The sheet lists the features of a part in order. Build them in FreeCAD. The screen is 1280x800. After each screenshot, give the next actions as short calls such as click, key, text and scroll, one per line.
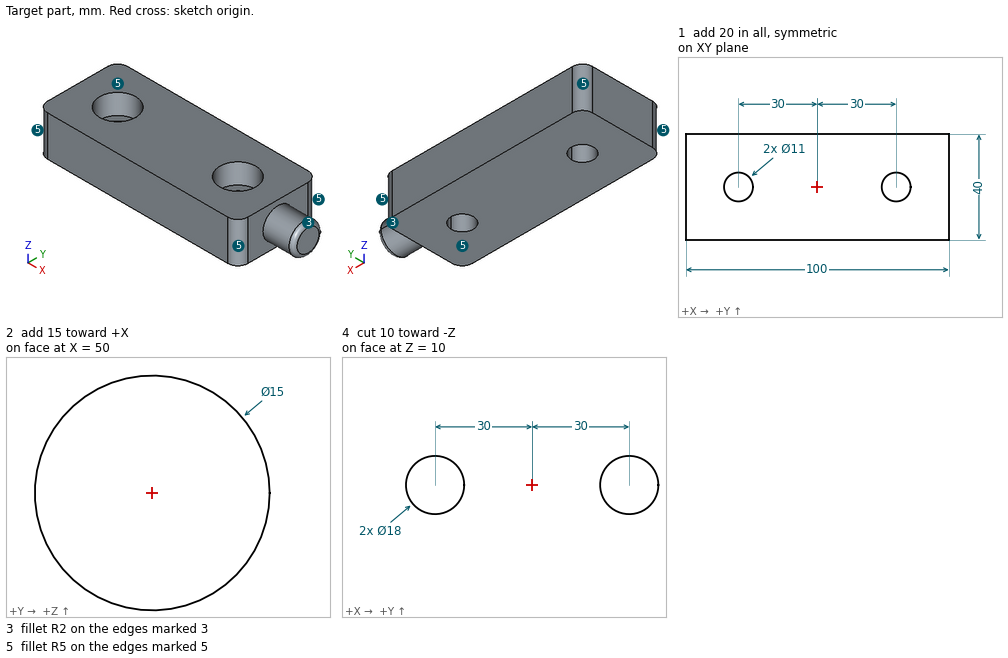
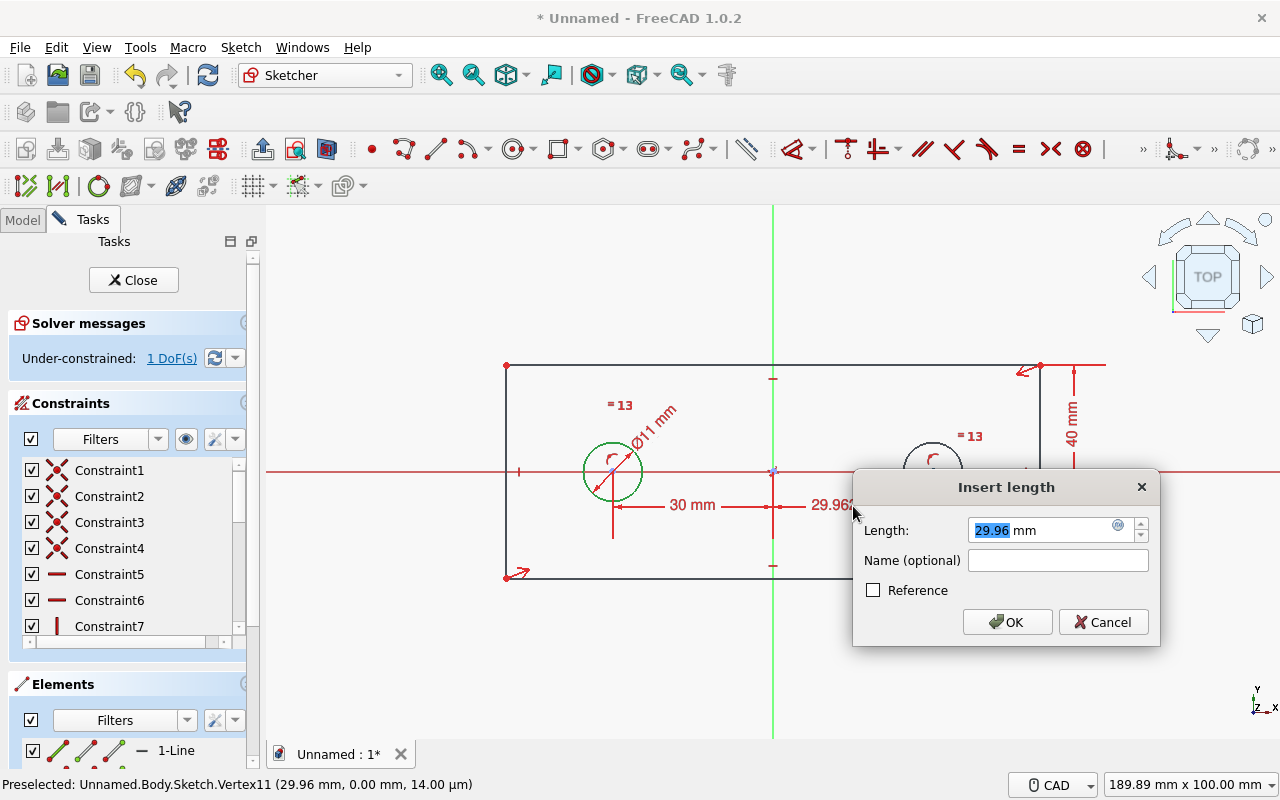
text(30)
key(Return)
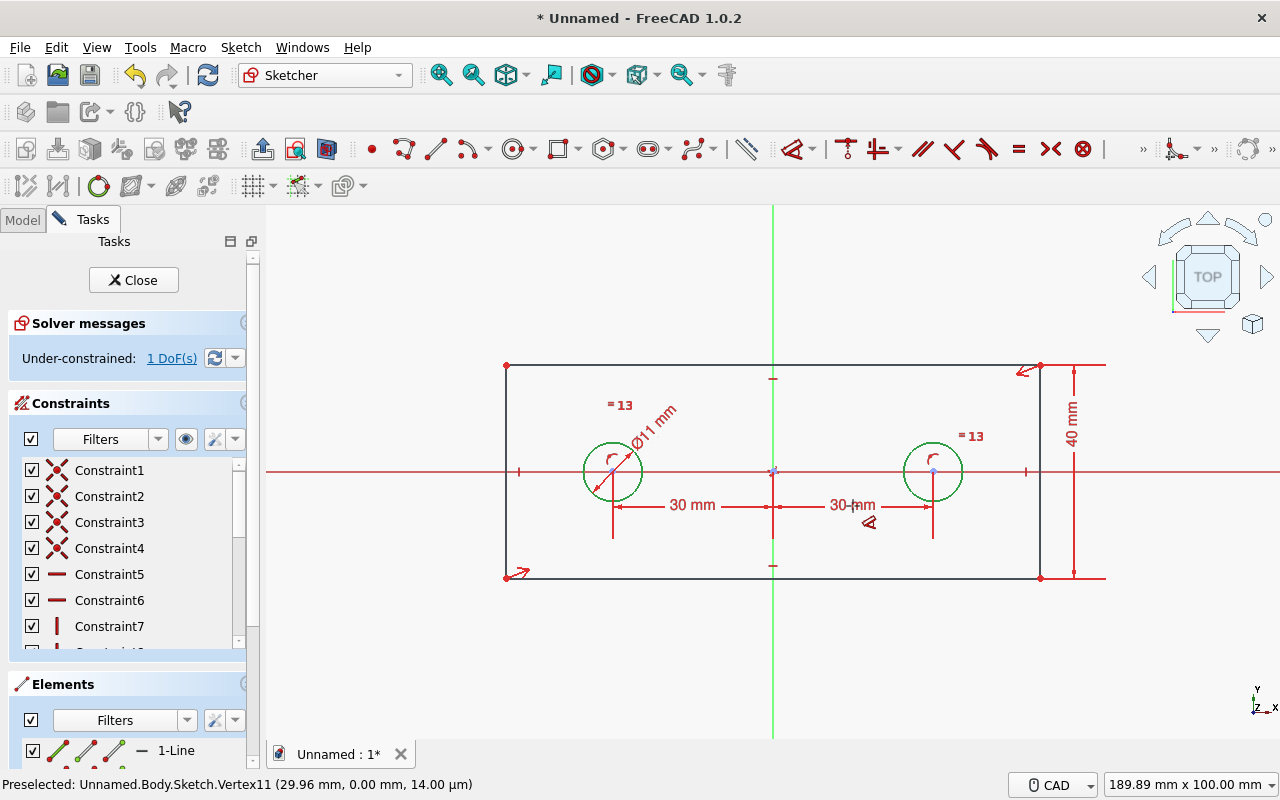
click(666, 579)
click(650, 613)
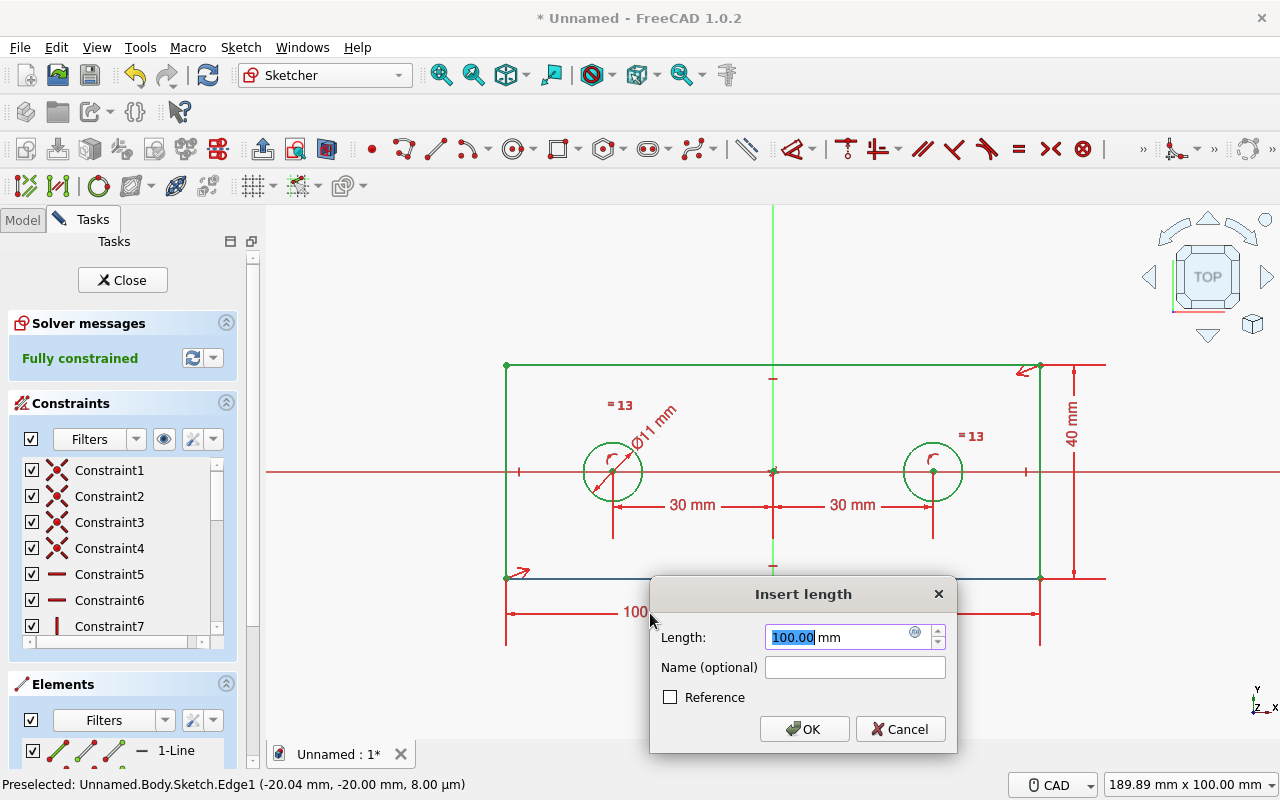
text(100)
key(Return)
key(Escape)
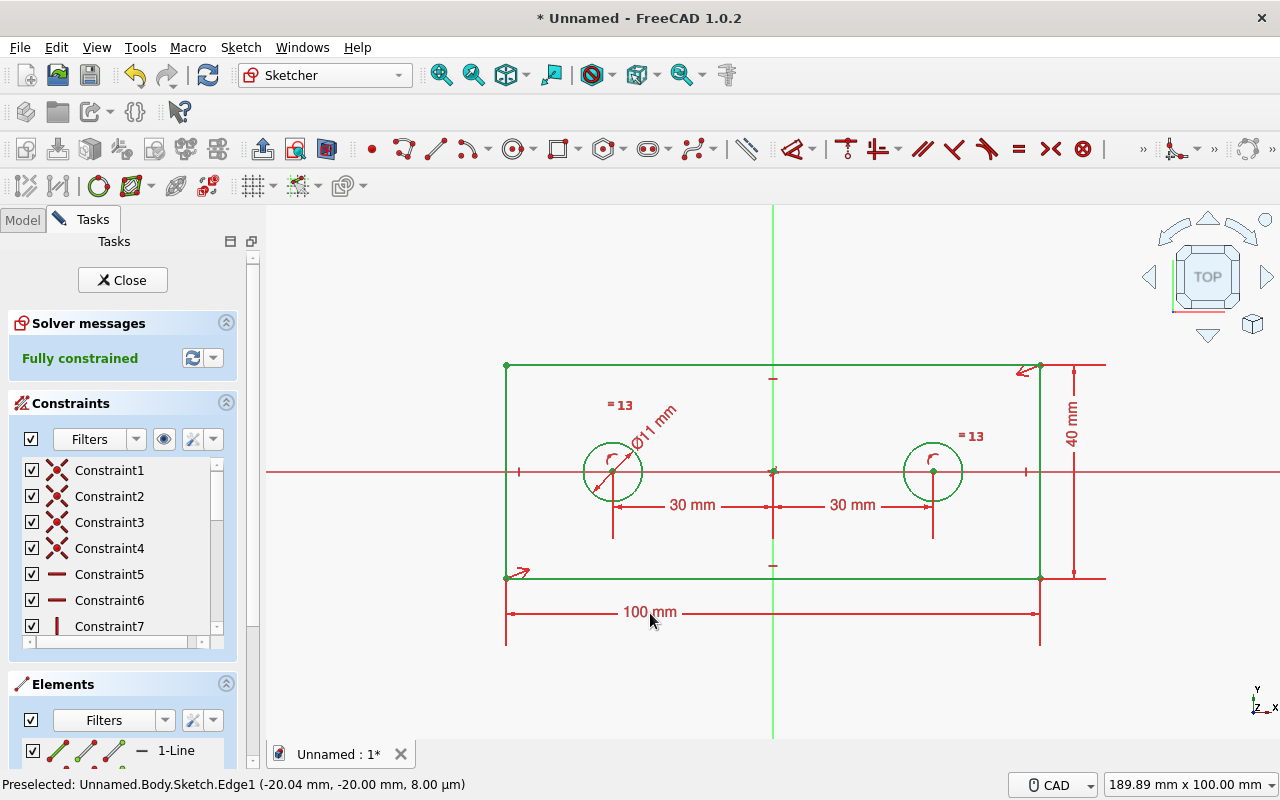
click(123, 280)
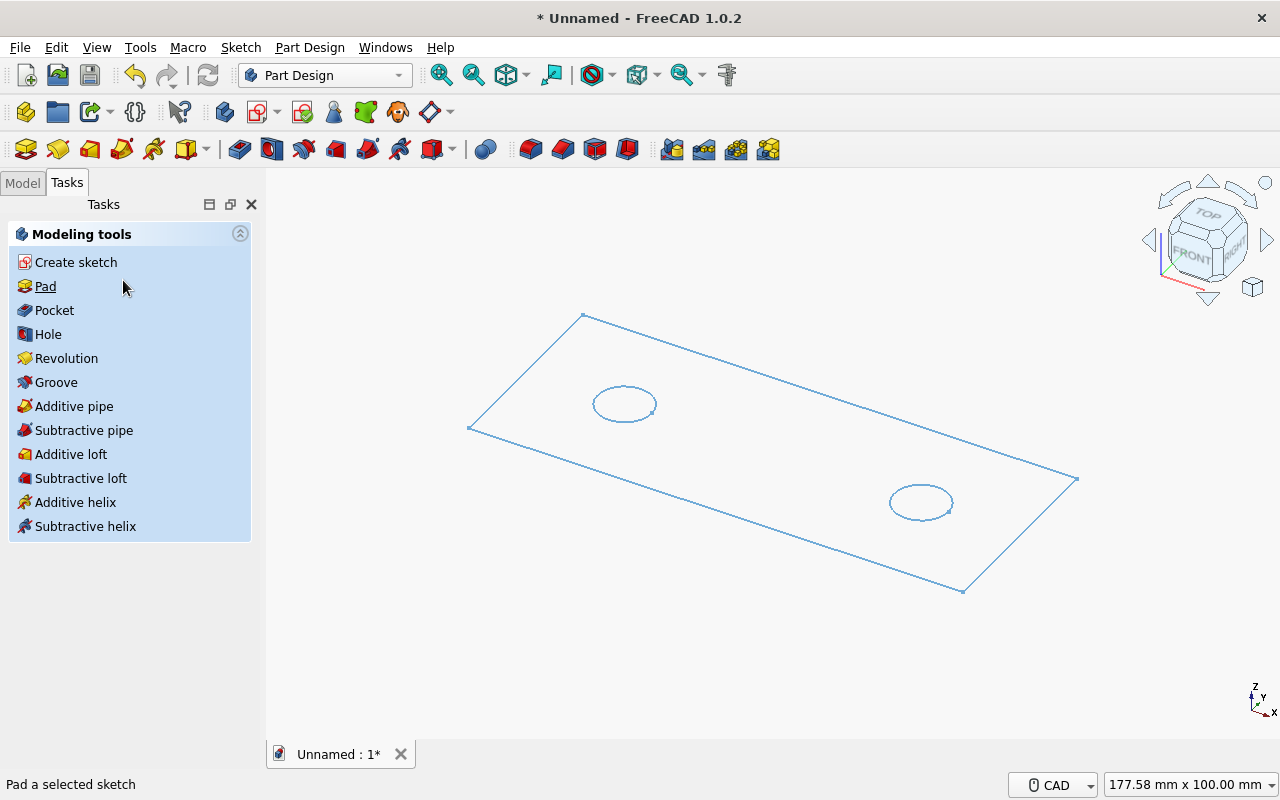
click(26, 150)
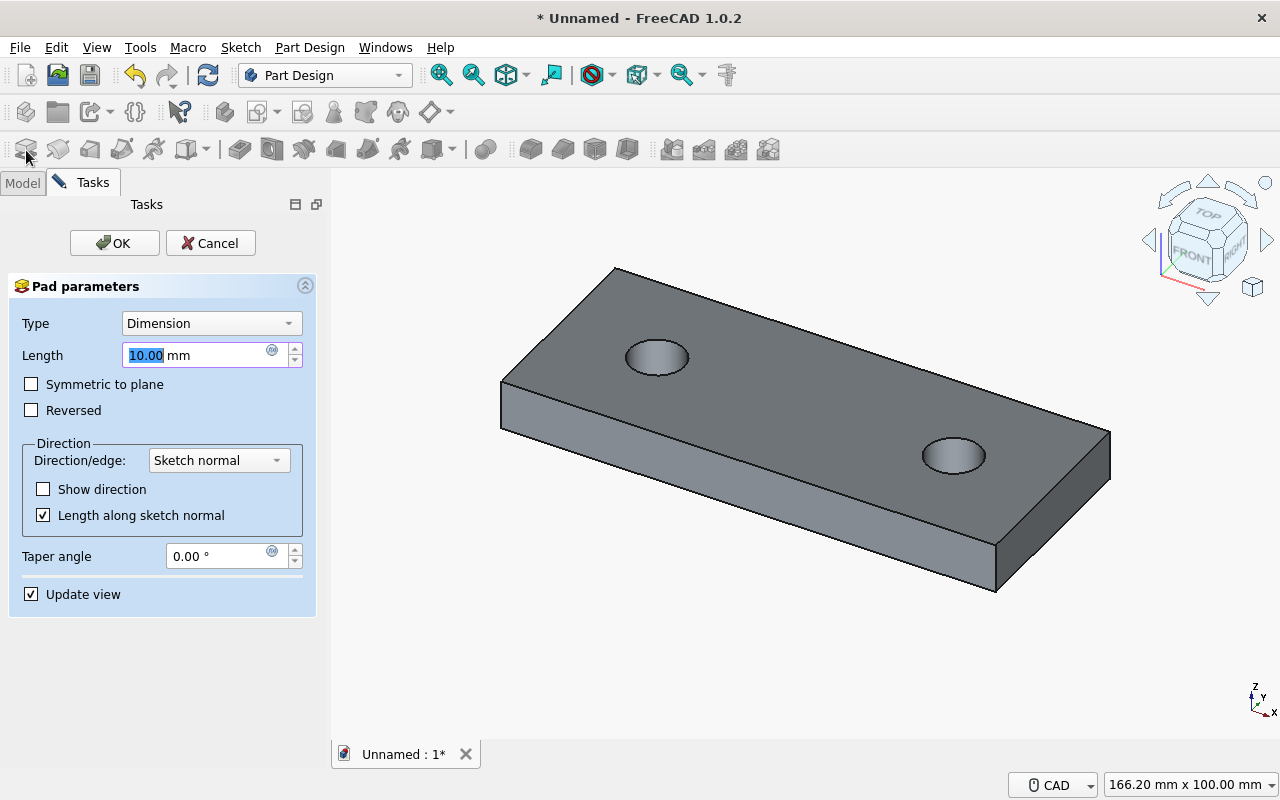
text(20)
key(Tab)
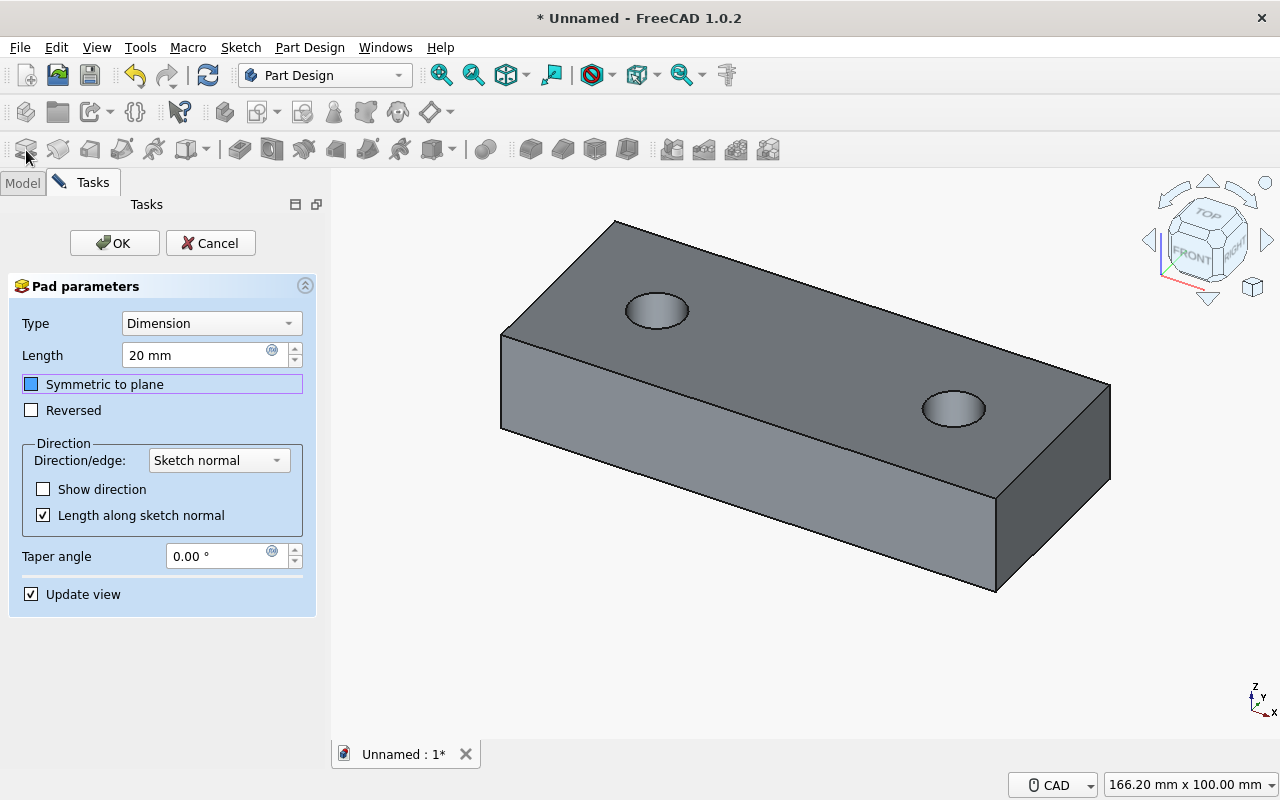
click(30, 384)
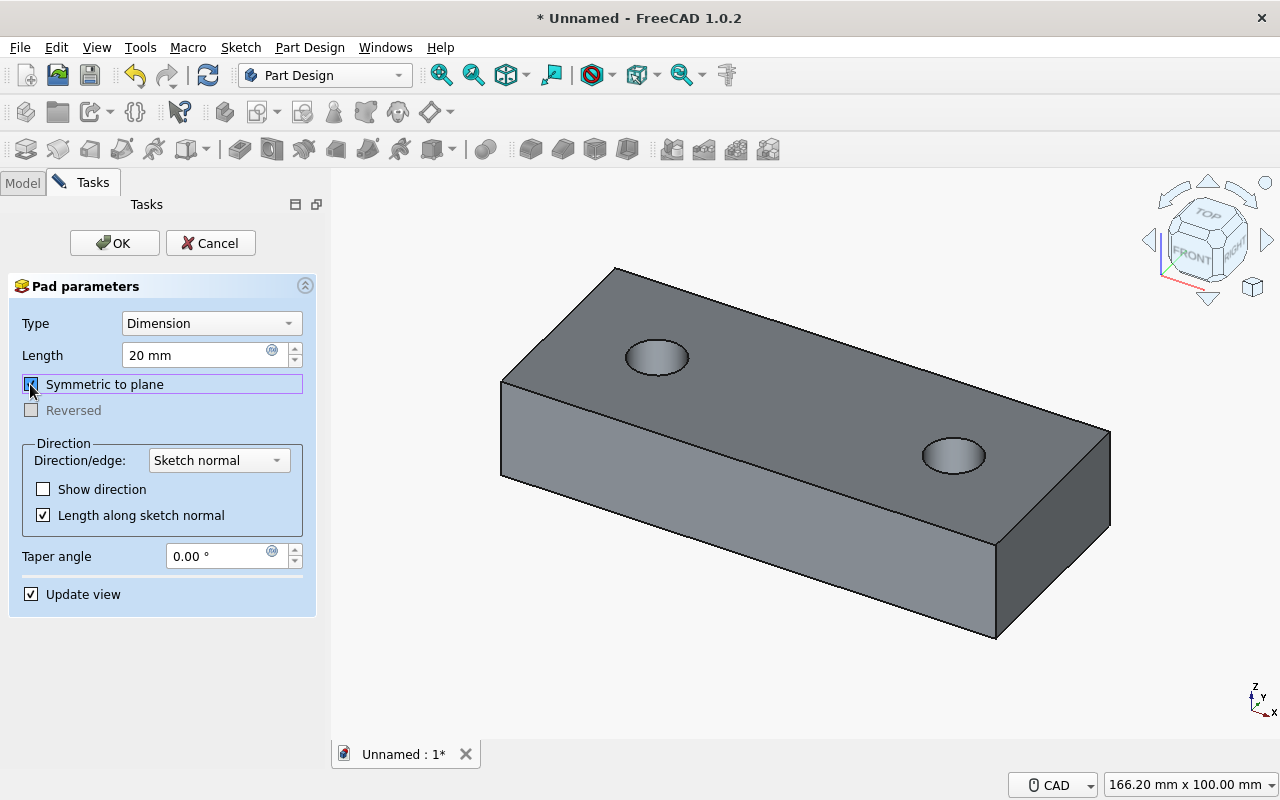
click(115, 243)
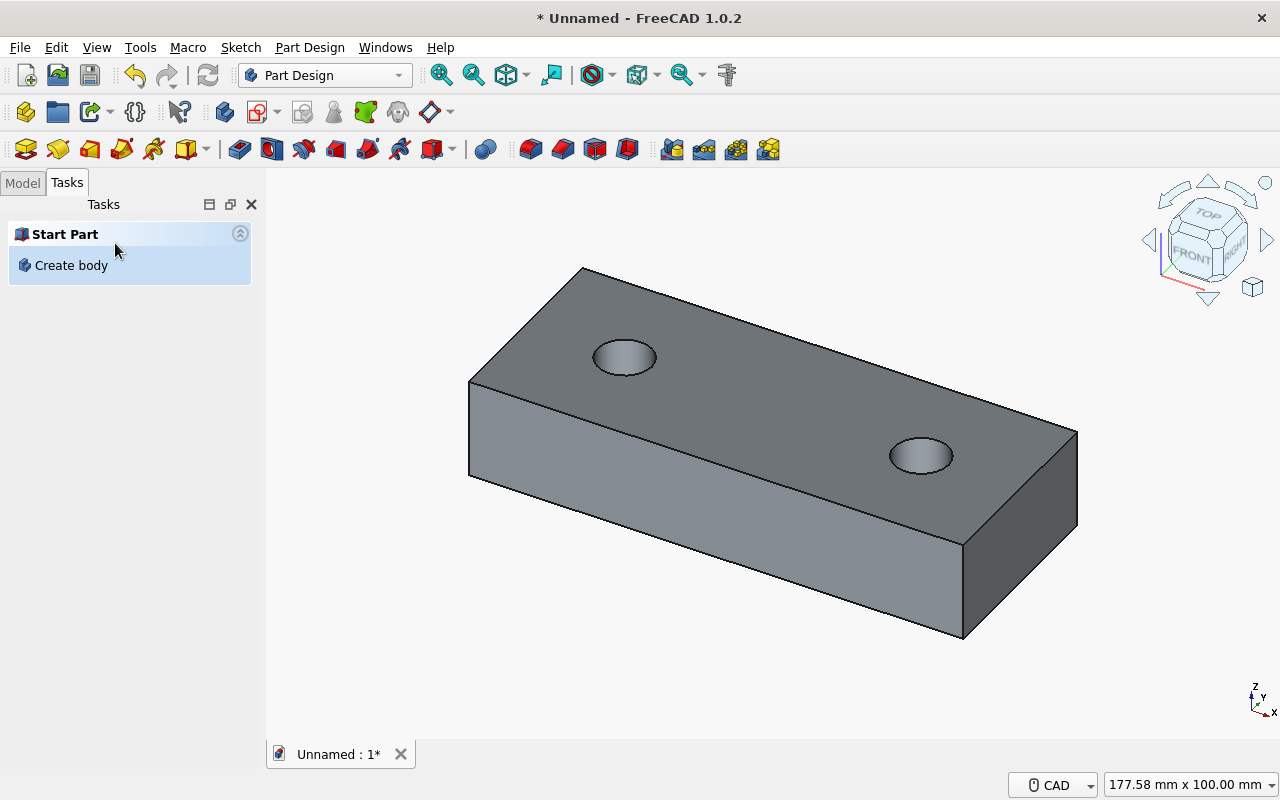
click(1037, 518)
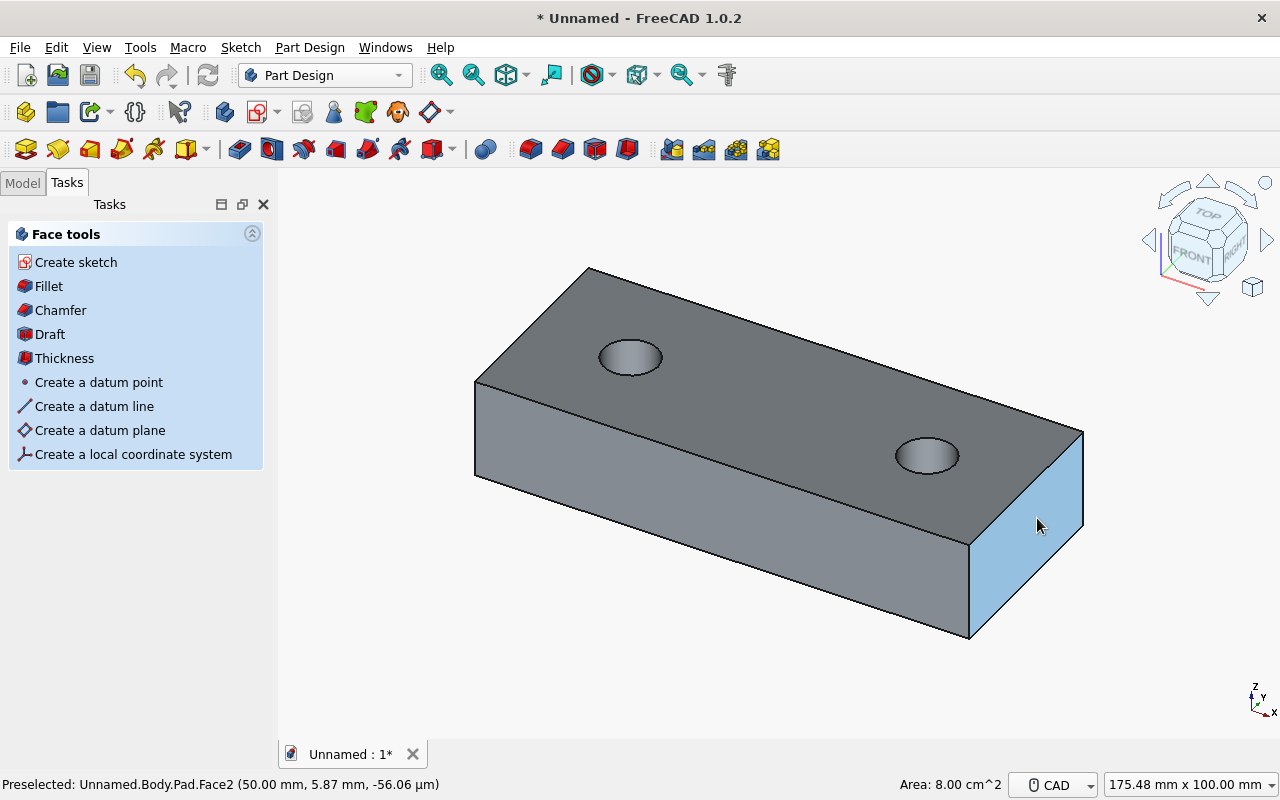
click(258, 112)